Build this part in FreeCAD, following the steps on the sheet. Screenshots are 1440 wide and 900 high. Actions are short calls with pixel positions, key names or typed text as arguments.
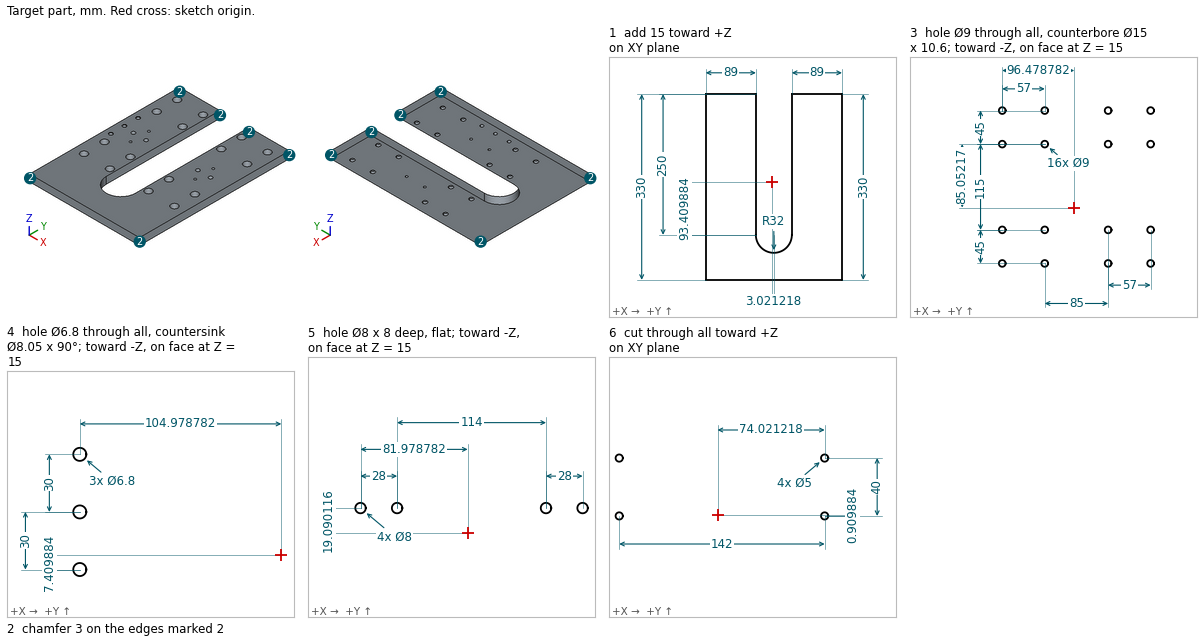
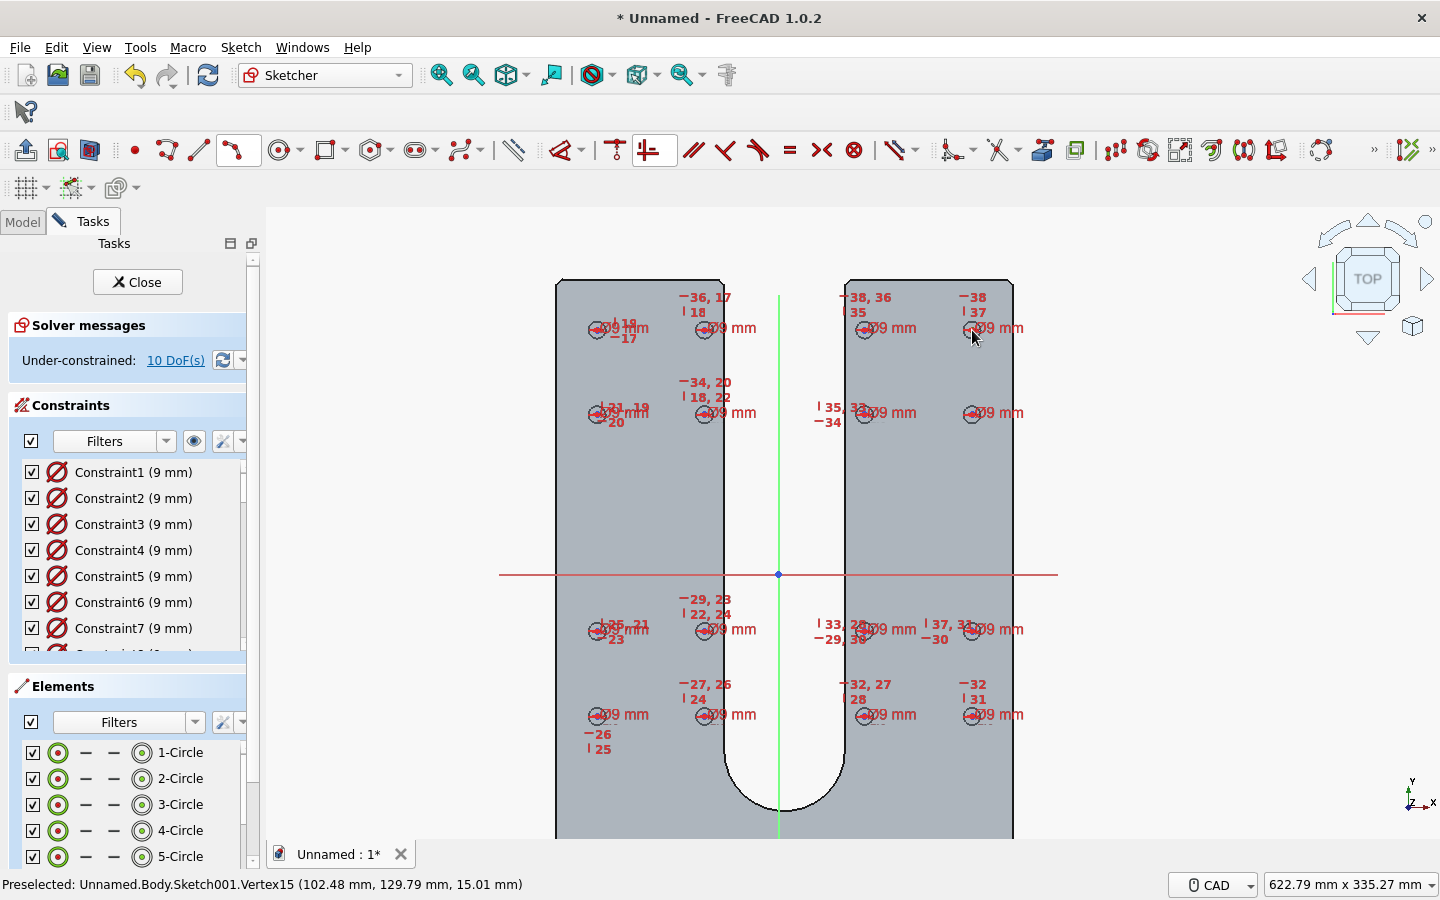
click(972, 415)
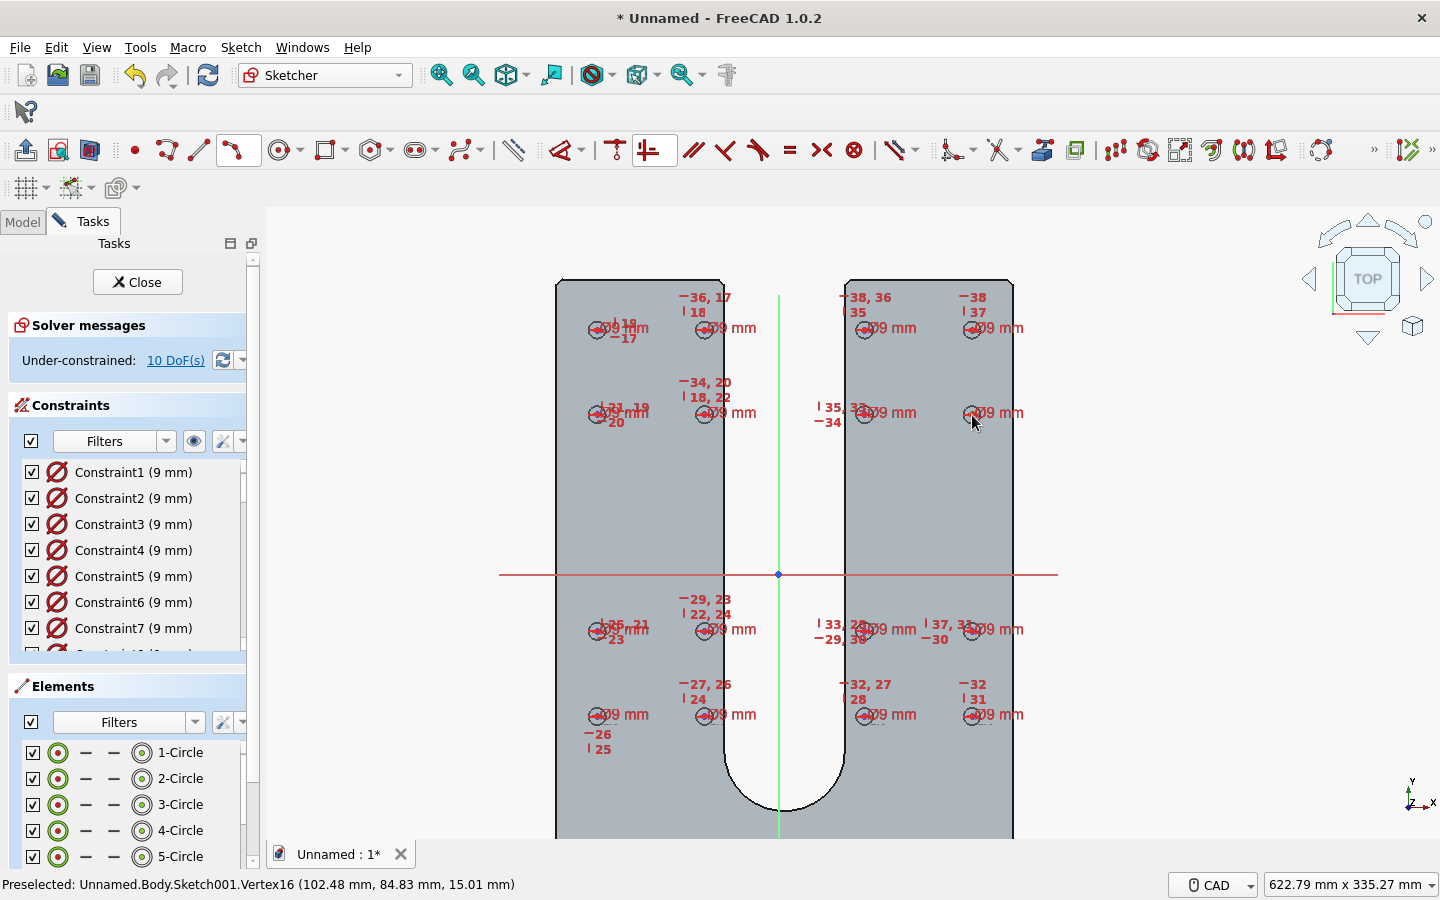
key(v)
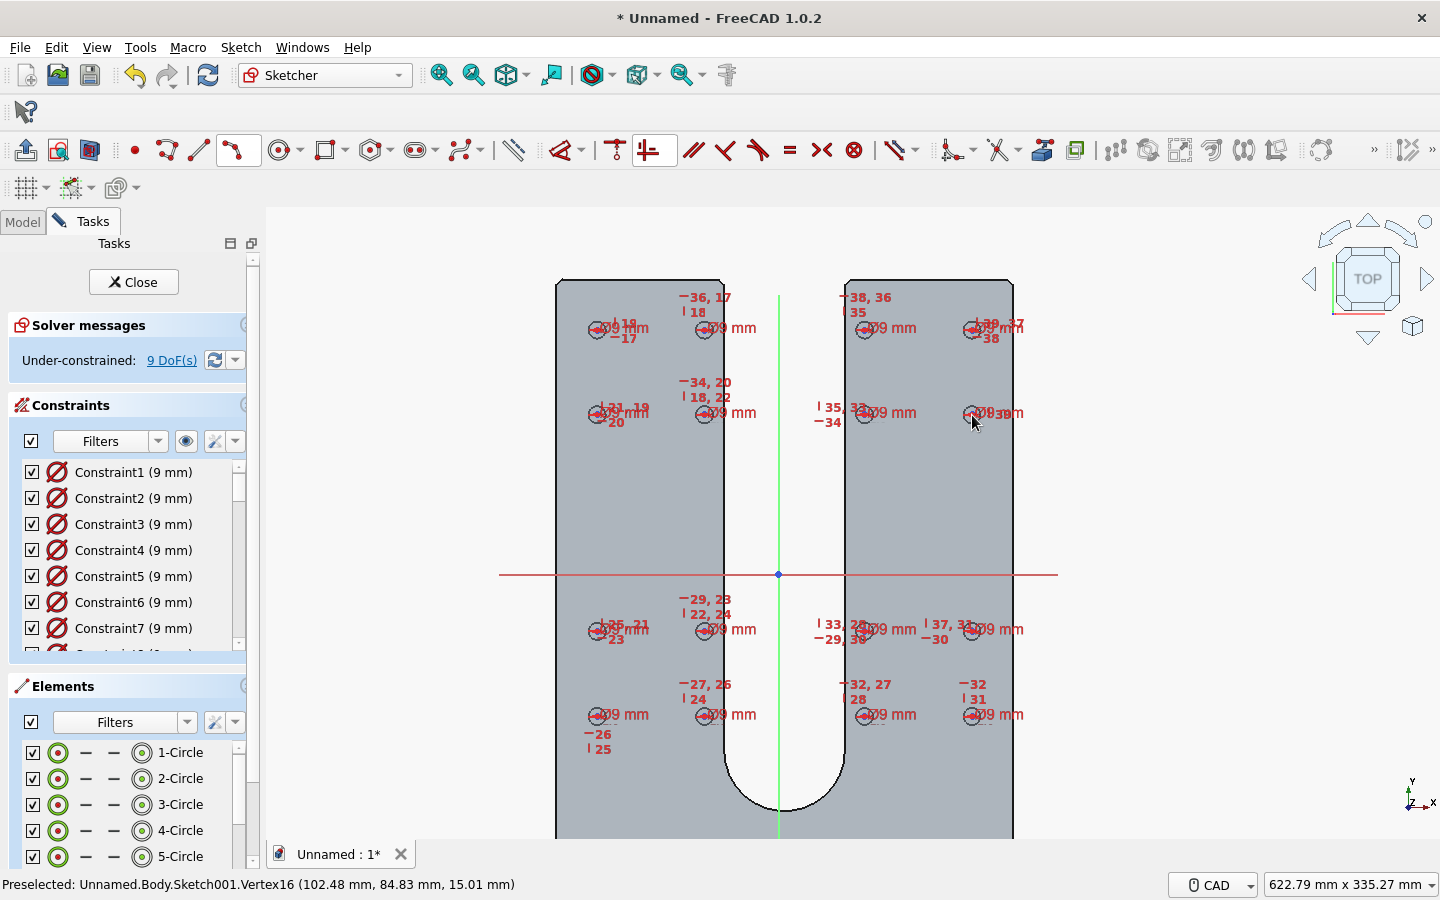
click(865, 415)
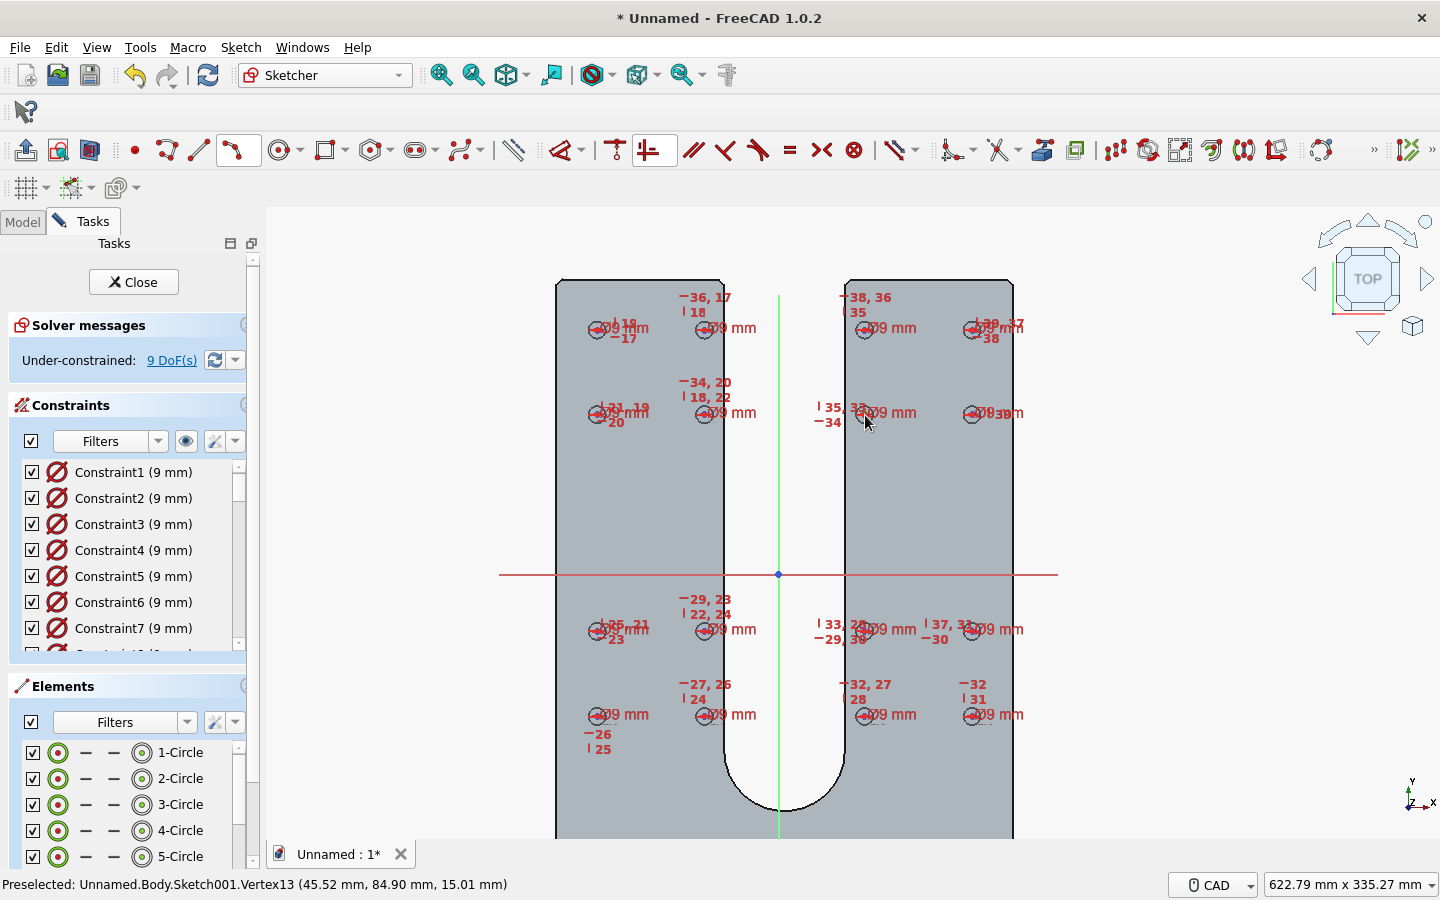
click(972, 415)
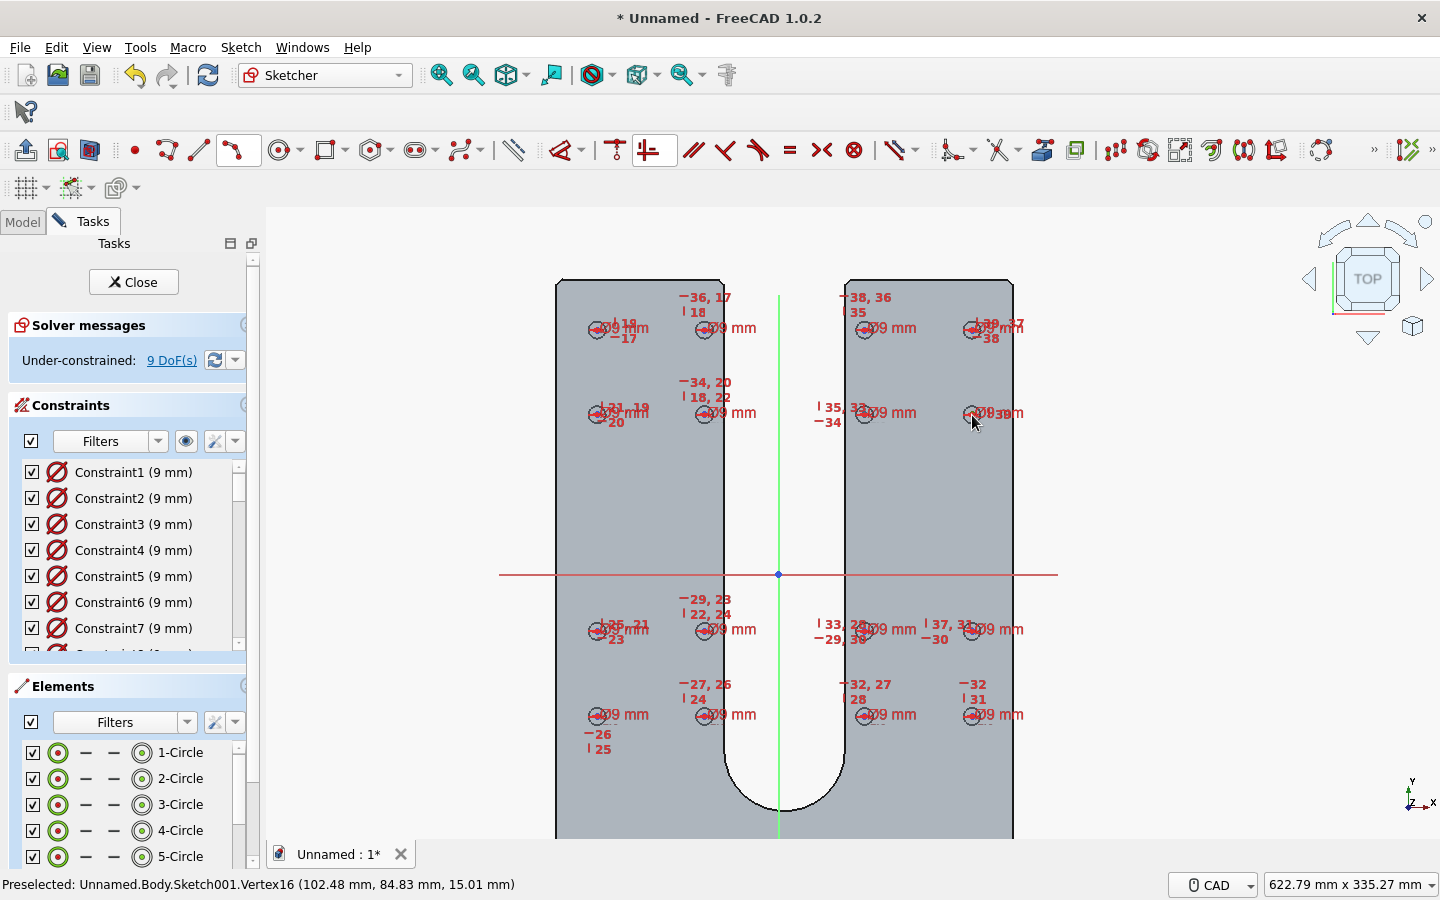
key(h)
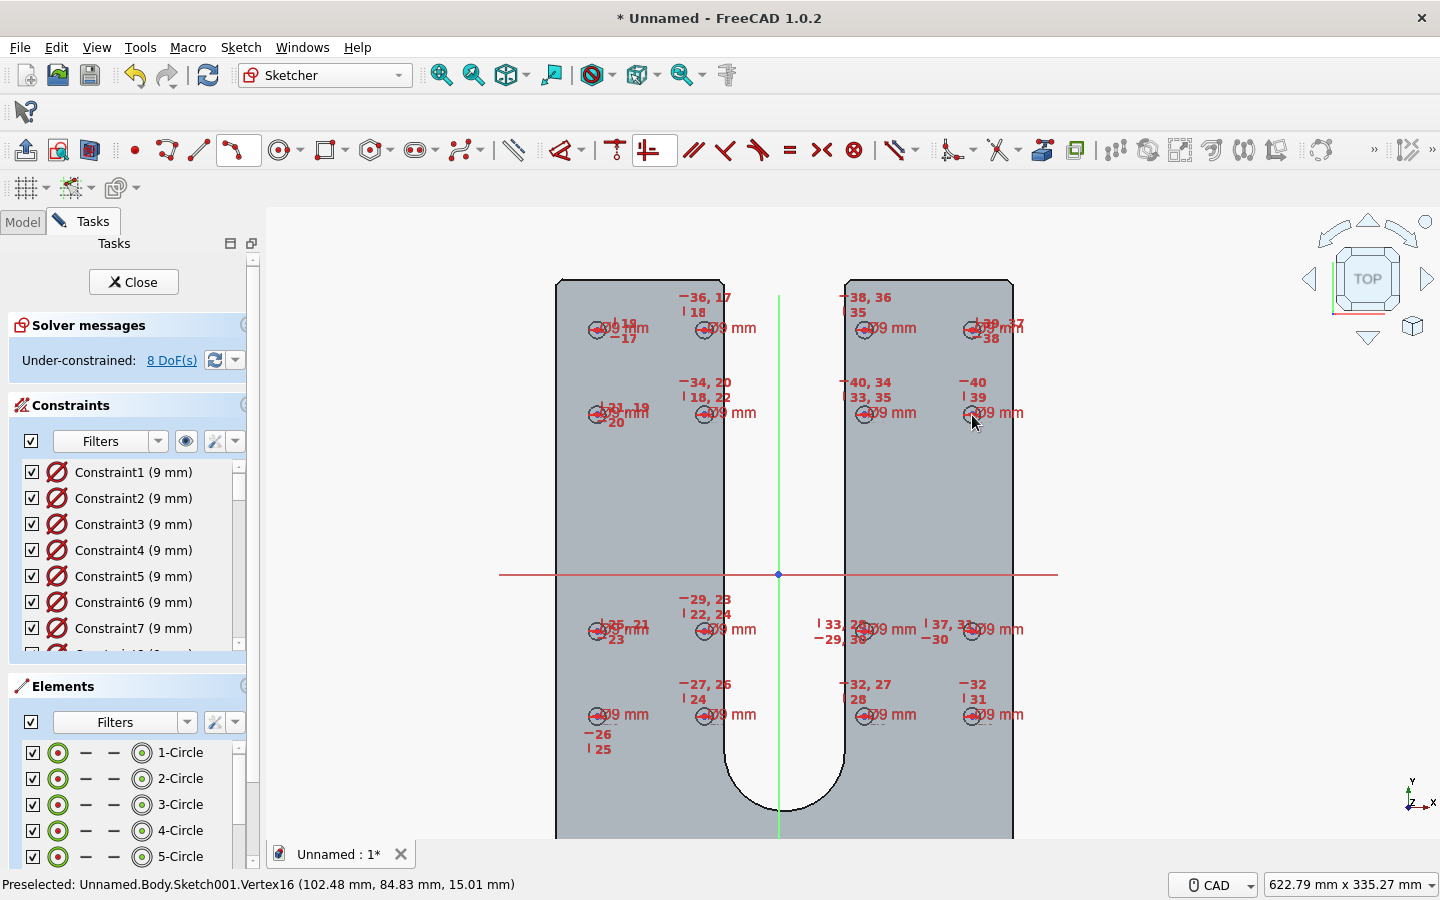
click(560, 150)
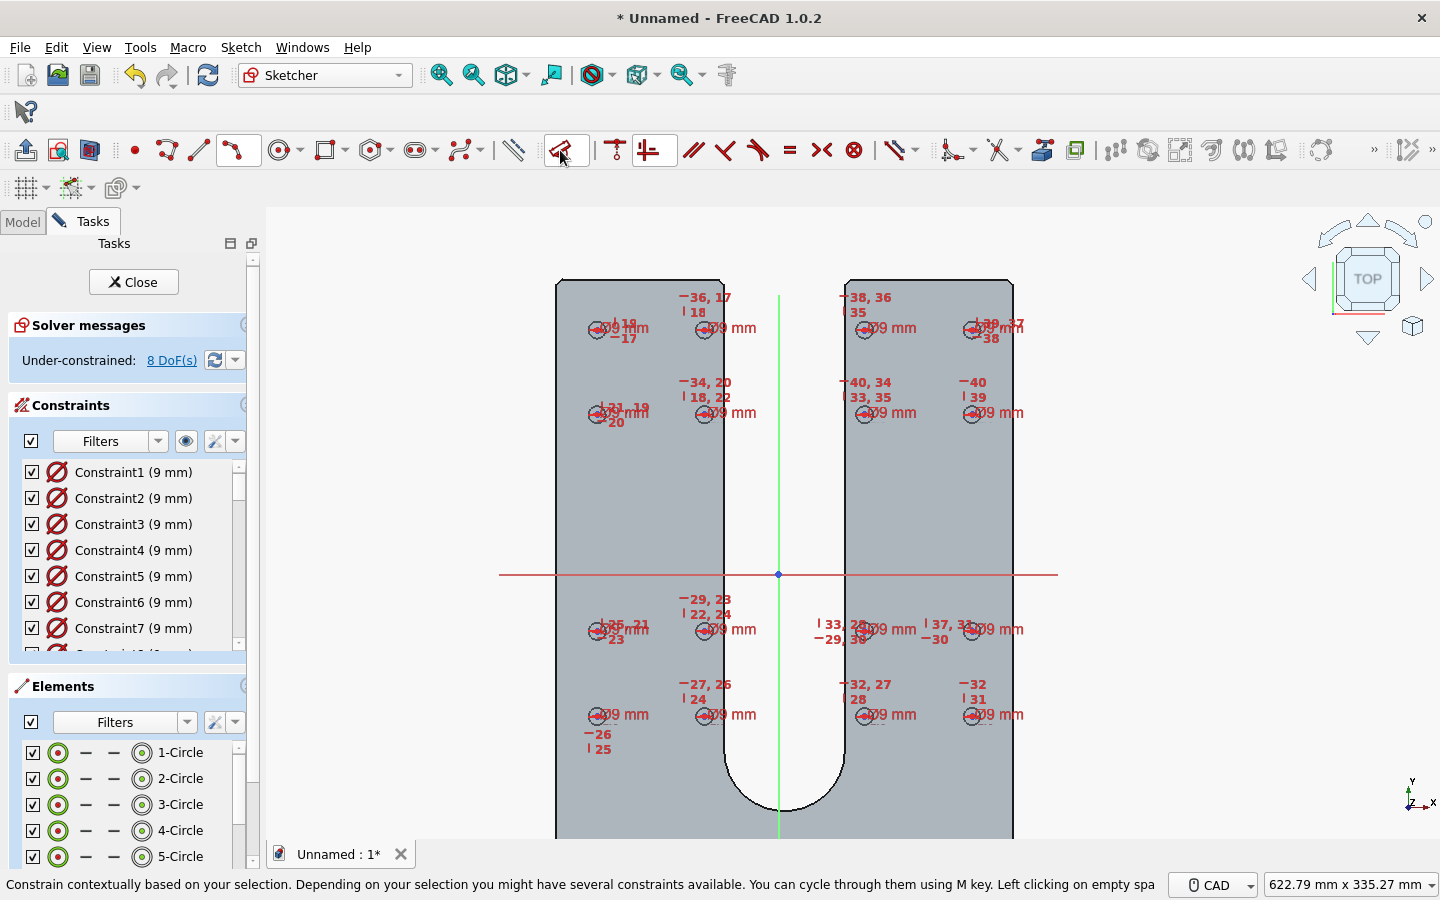
click(597, 330)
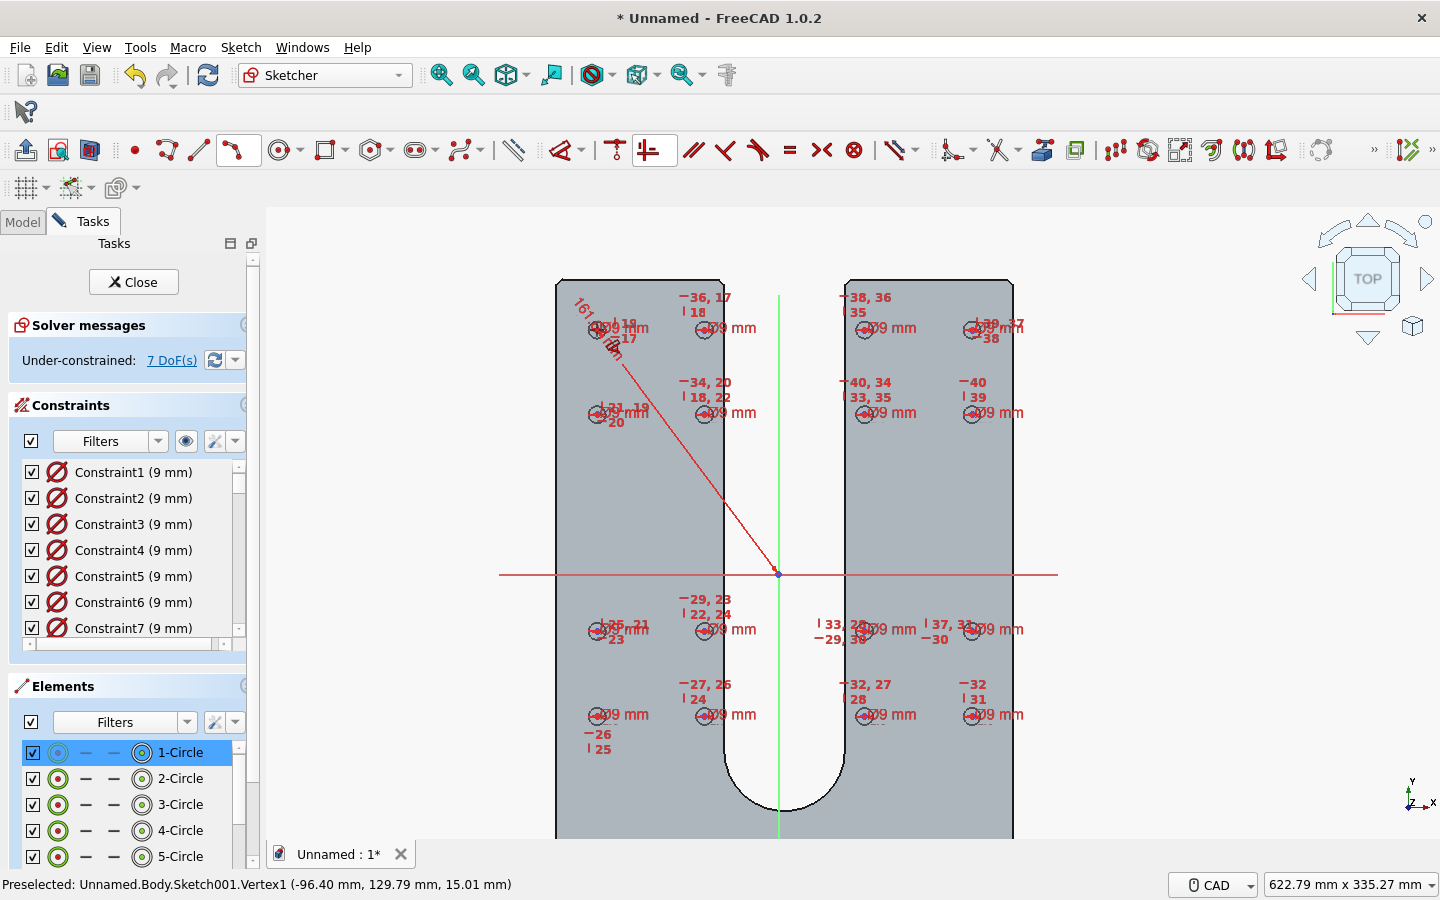
click(705, 330)
click(651, 296)